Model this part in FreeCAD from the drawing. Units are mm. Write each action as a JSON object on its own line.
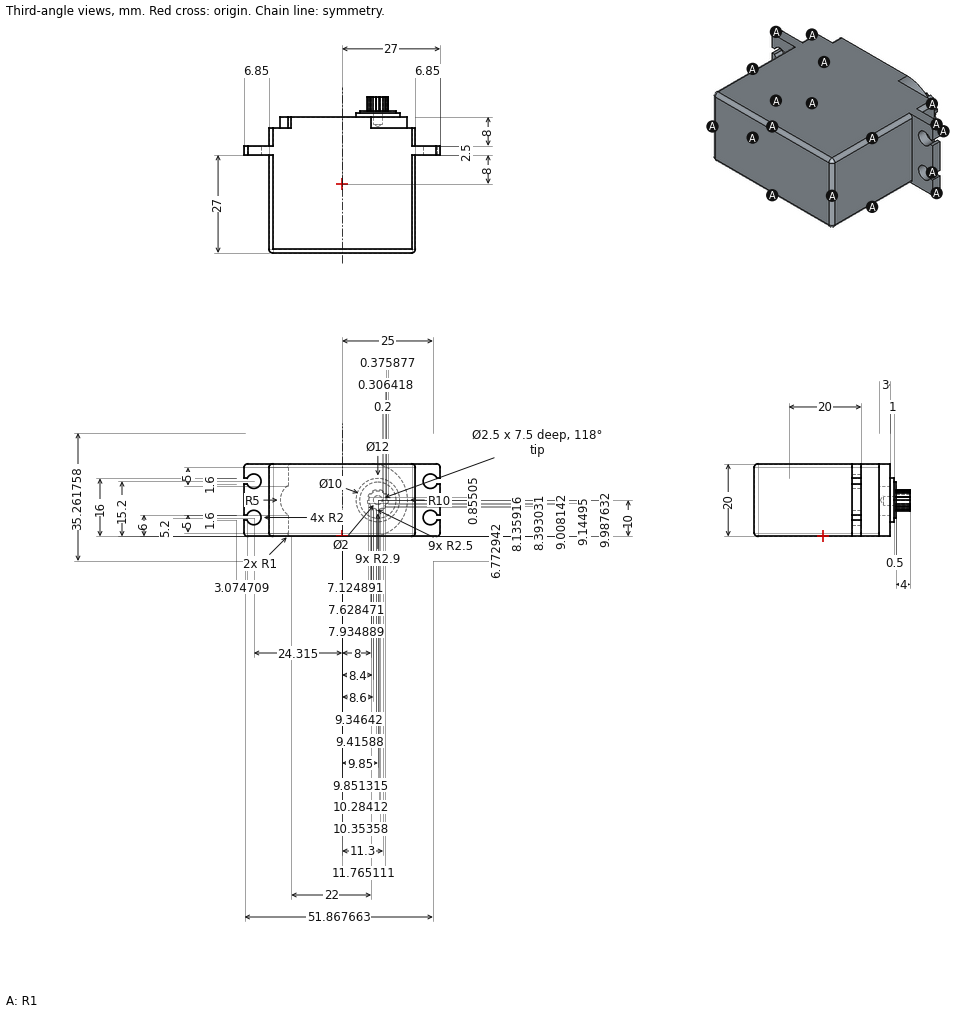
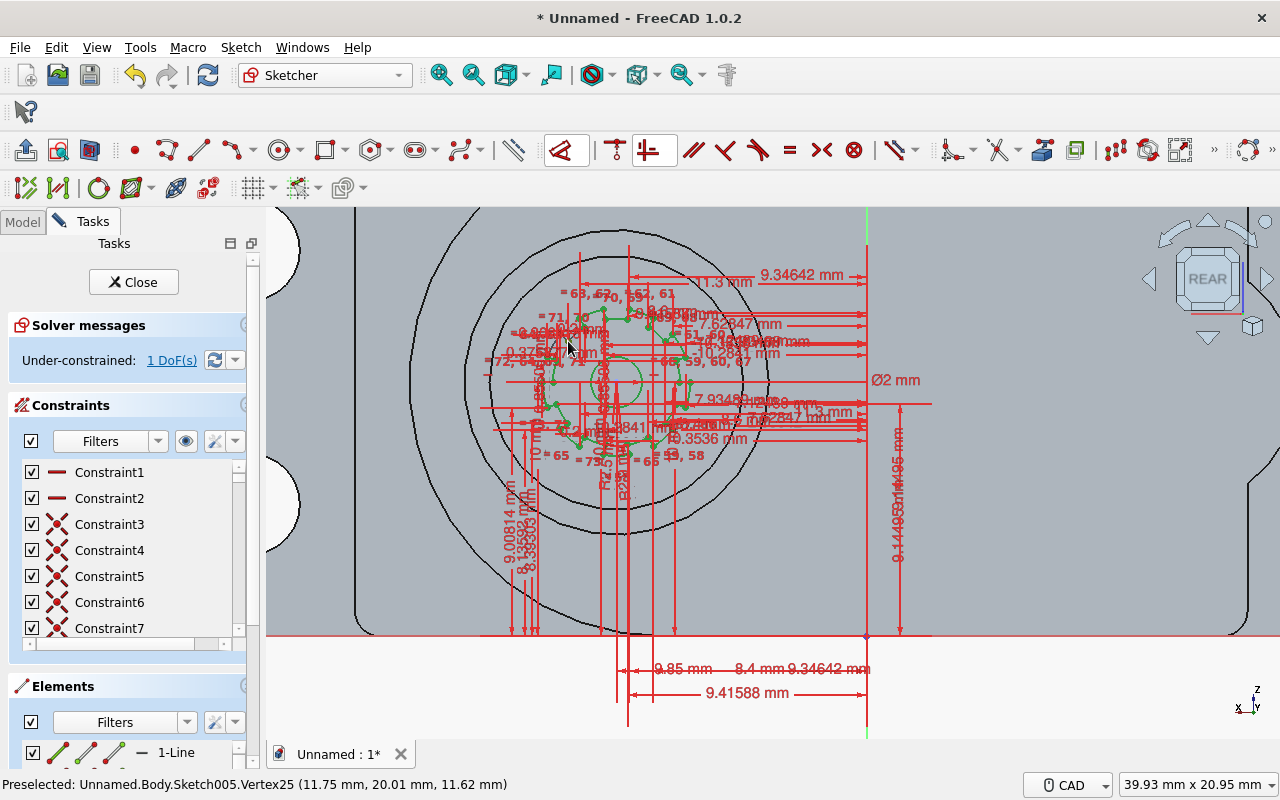
{"action": "left_click", "coordinate": [584, 150]}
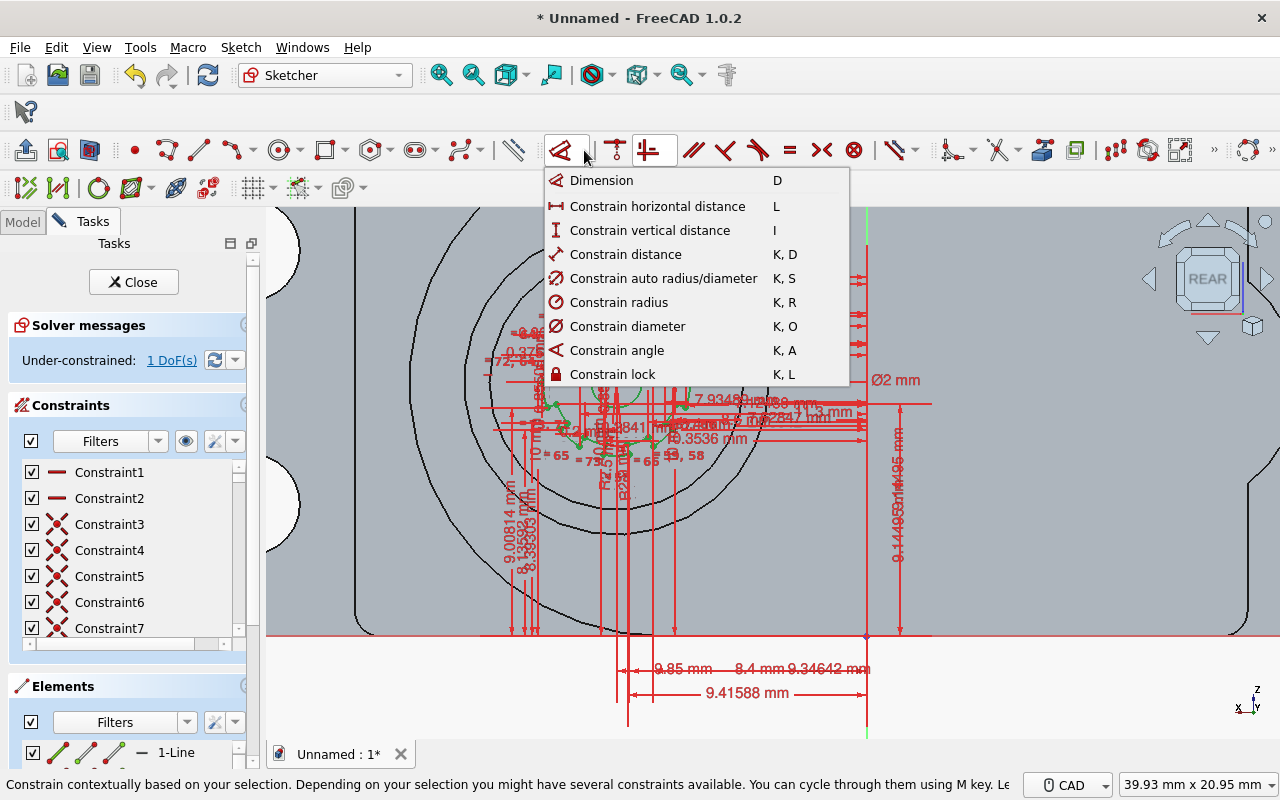
{"action": "left_click", "coordinate": [697, 206]}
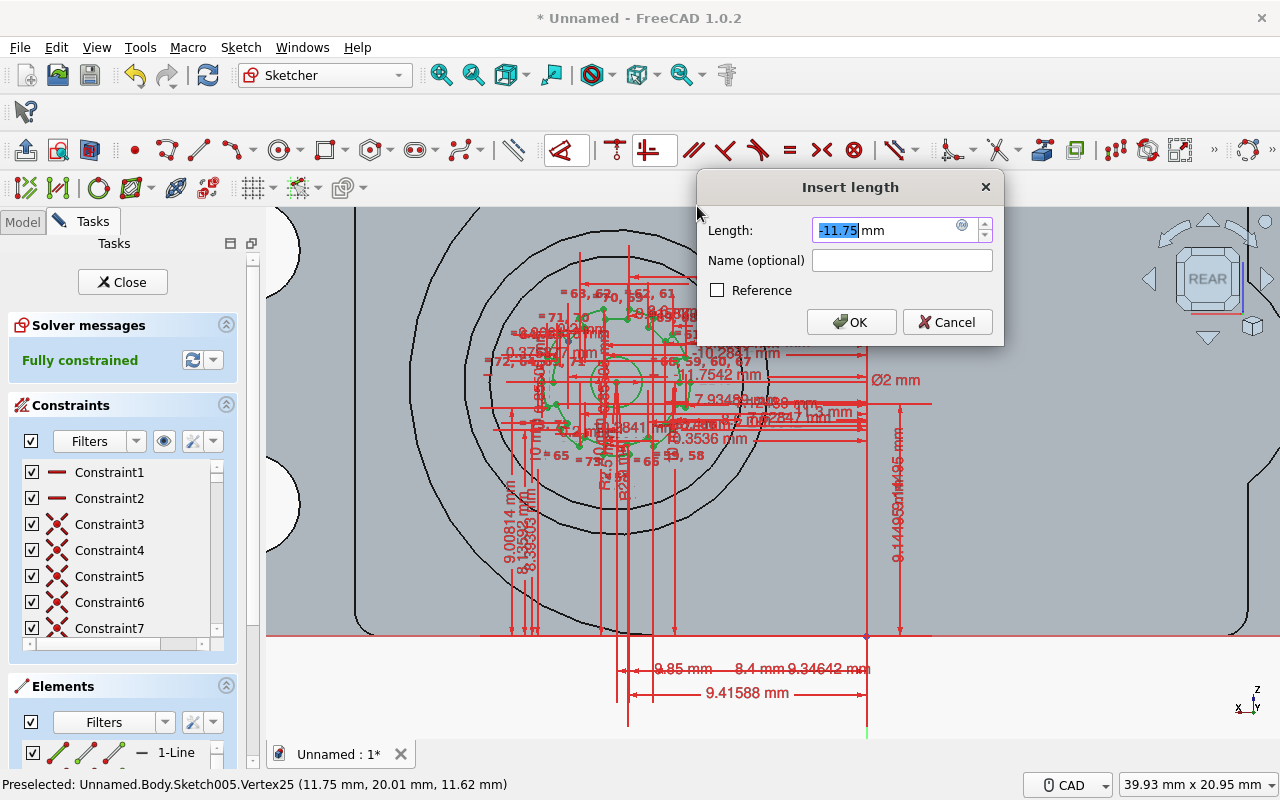
{"action": "type", "text": "-11.765111"}
{"action": "key", "text": "Return"}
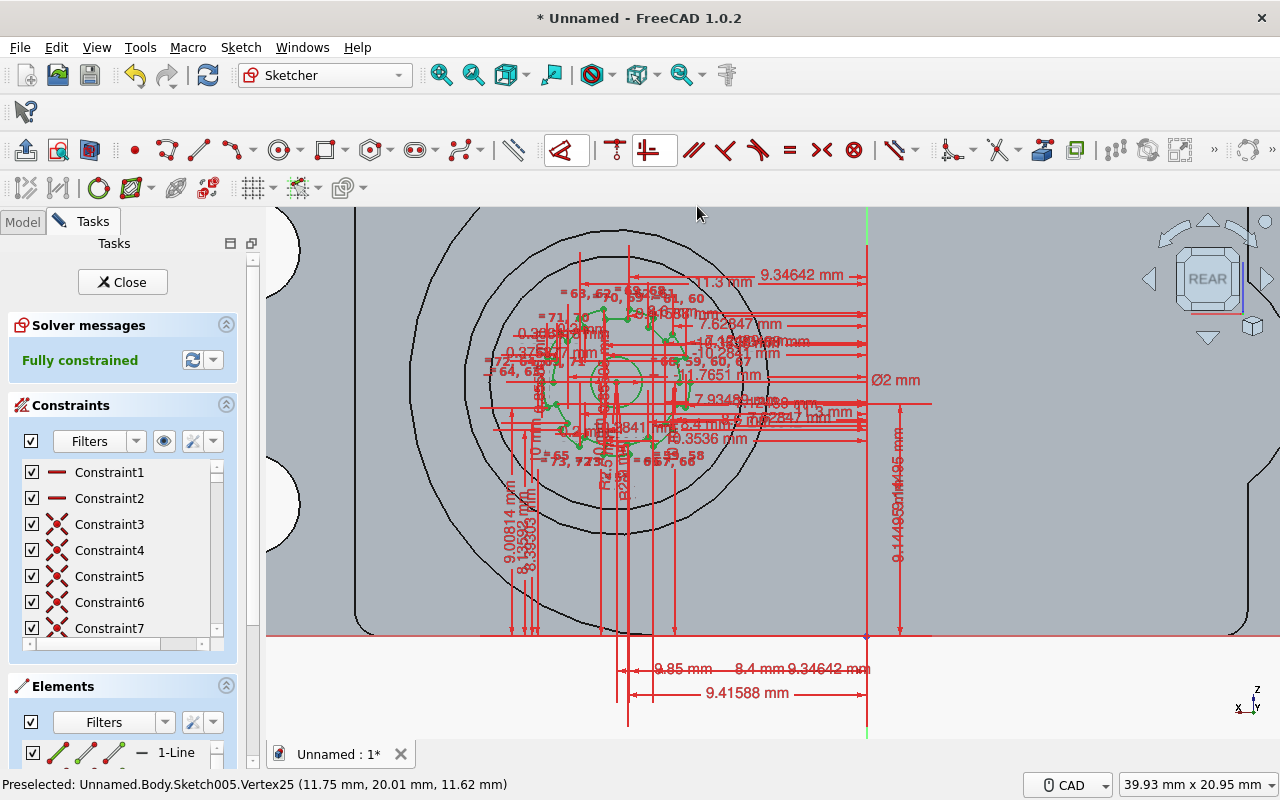
{"action": "left_click", "coordinate": [123, 282]}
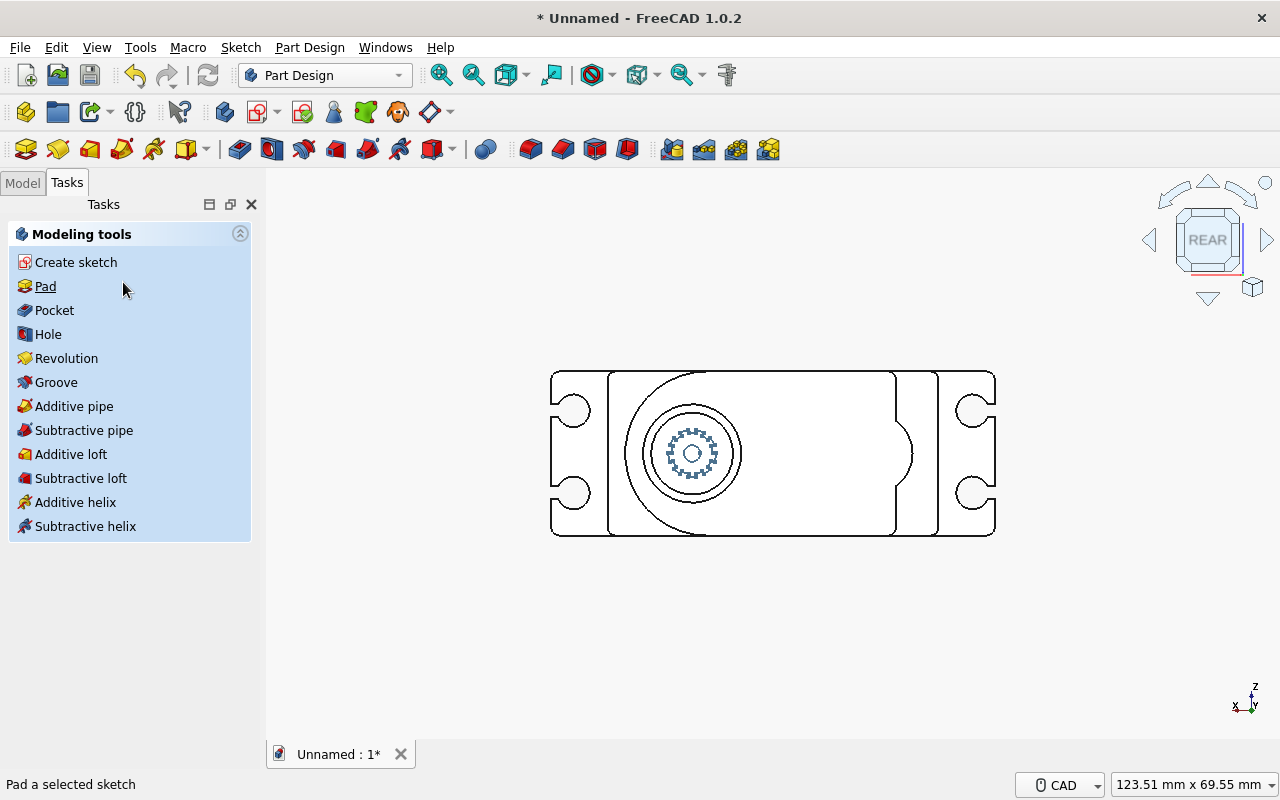
{"action": "left_click", "coordinate": [26, 150]}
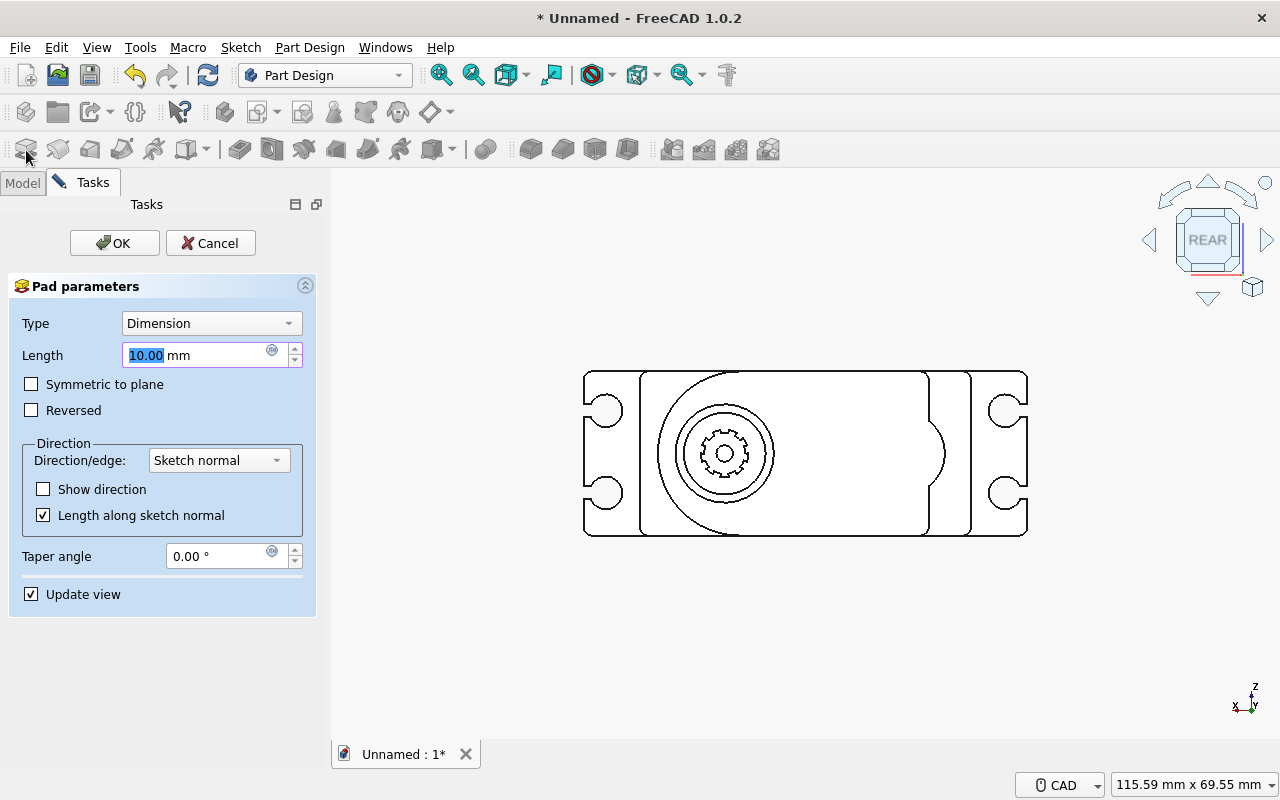
{"action": "type", "text": "4"}
{"action": "key", "text": "Tab"}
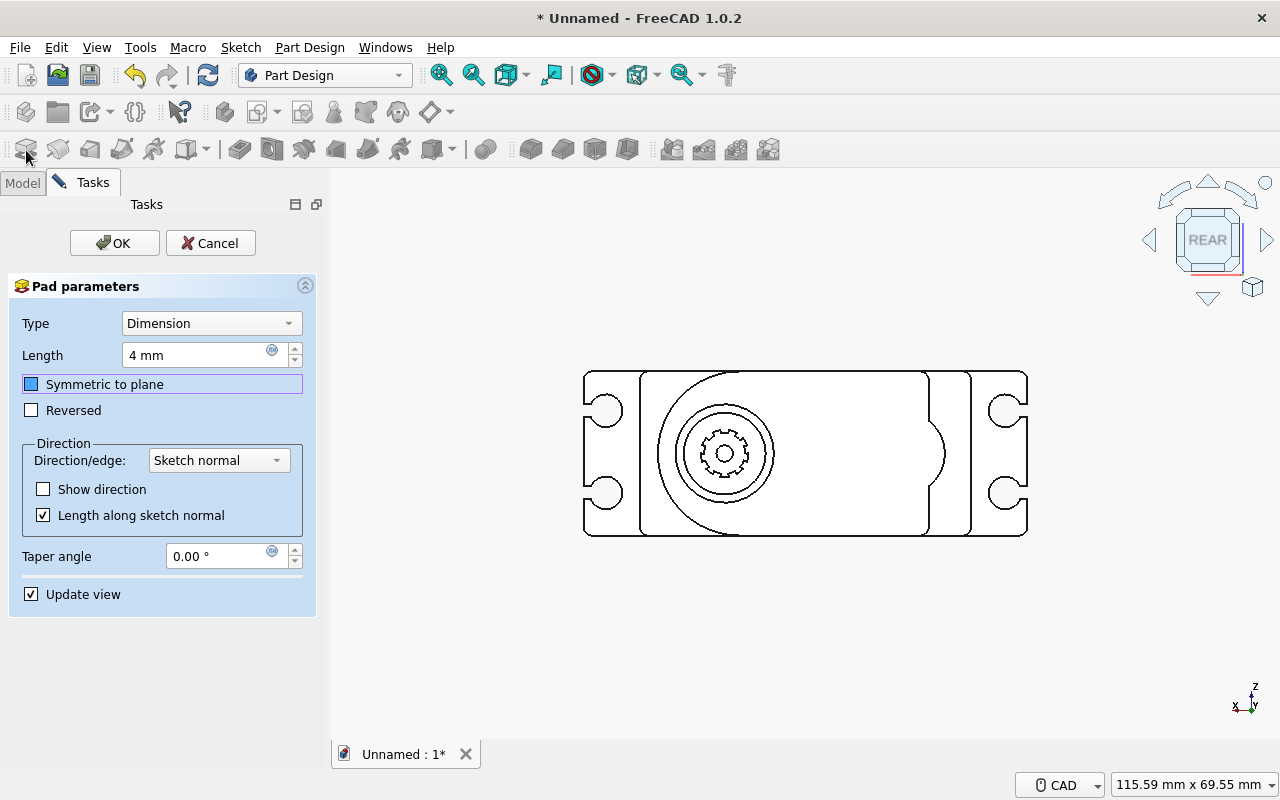
{"action": "left_click", "coordinate": [115, 243]}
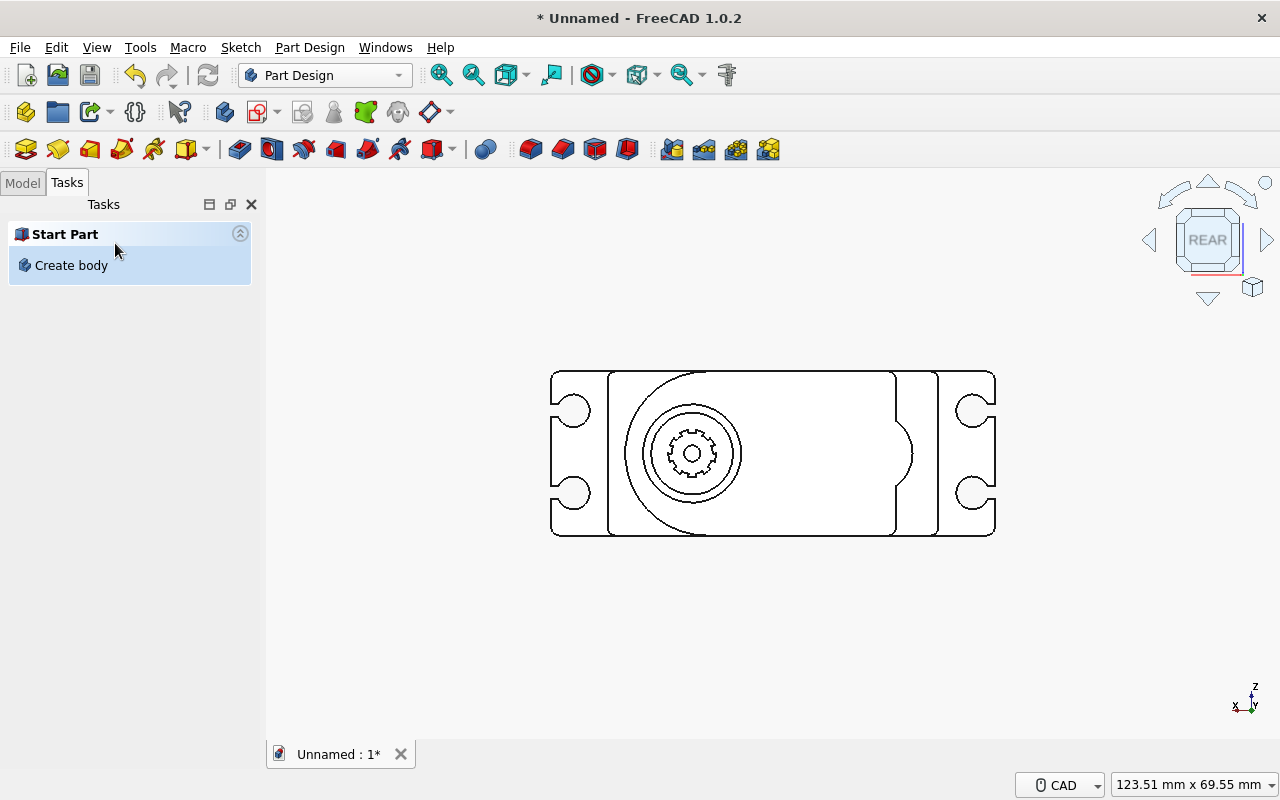
{"action": "key", "text": "v f"}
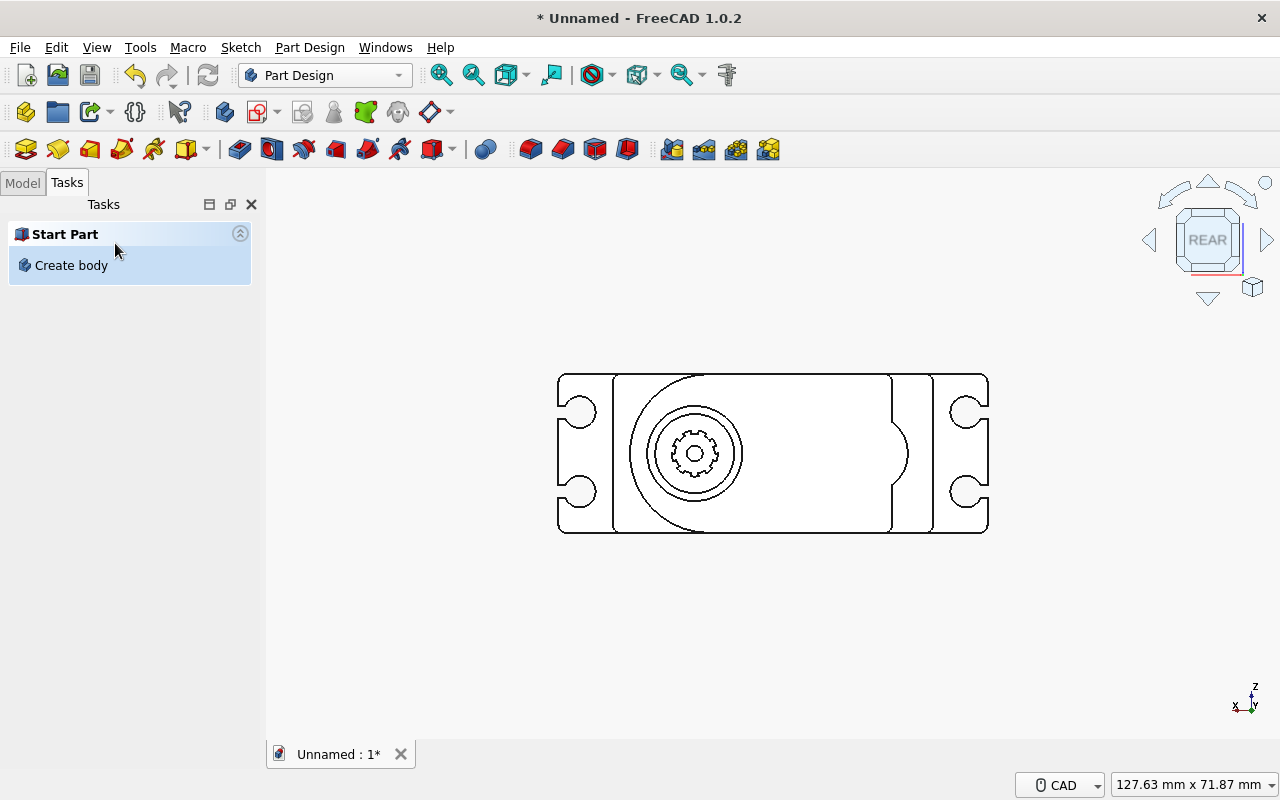
{"action": "scroll", "coordinate": [708, 446], "scroll_direction": "up", "scroll_amount": 4}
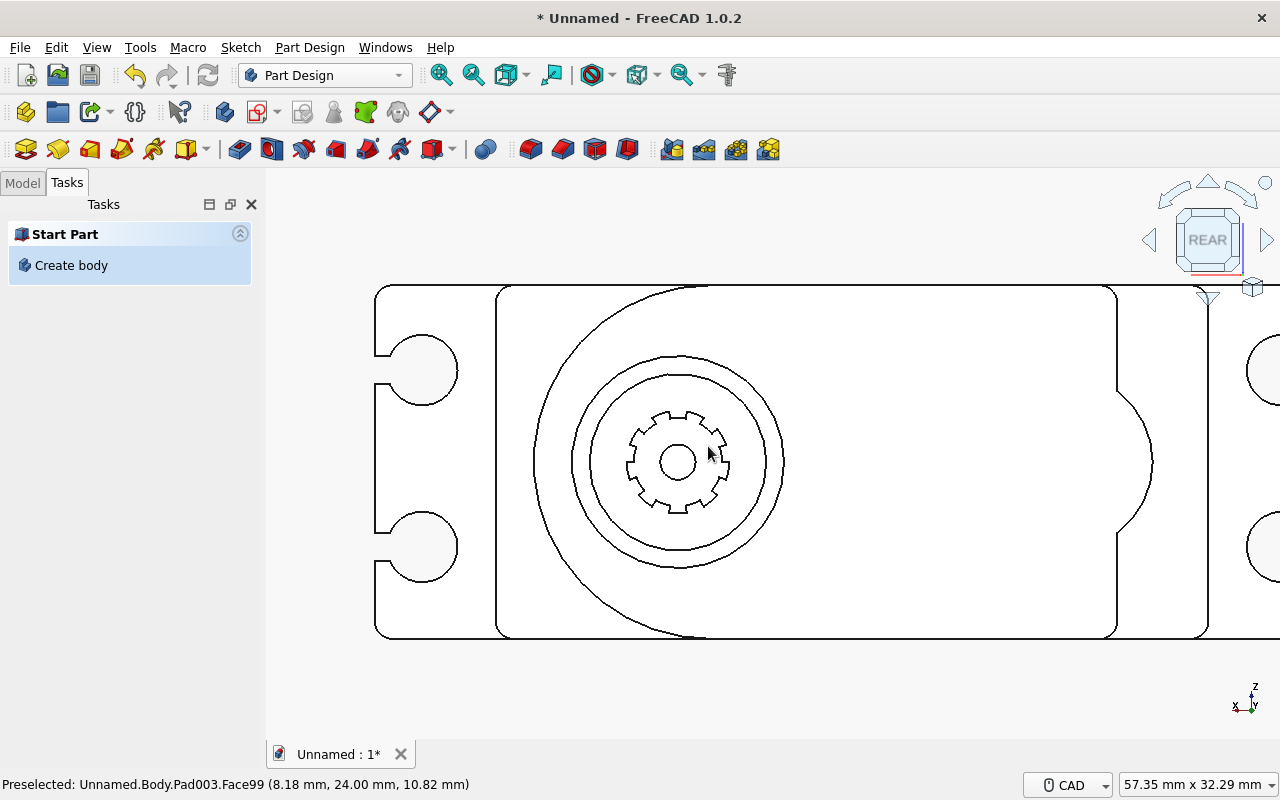
{"action": "left_click", "coordinate": [707, 447]}